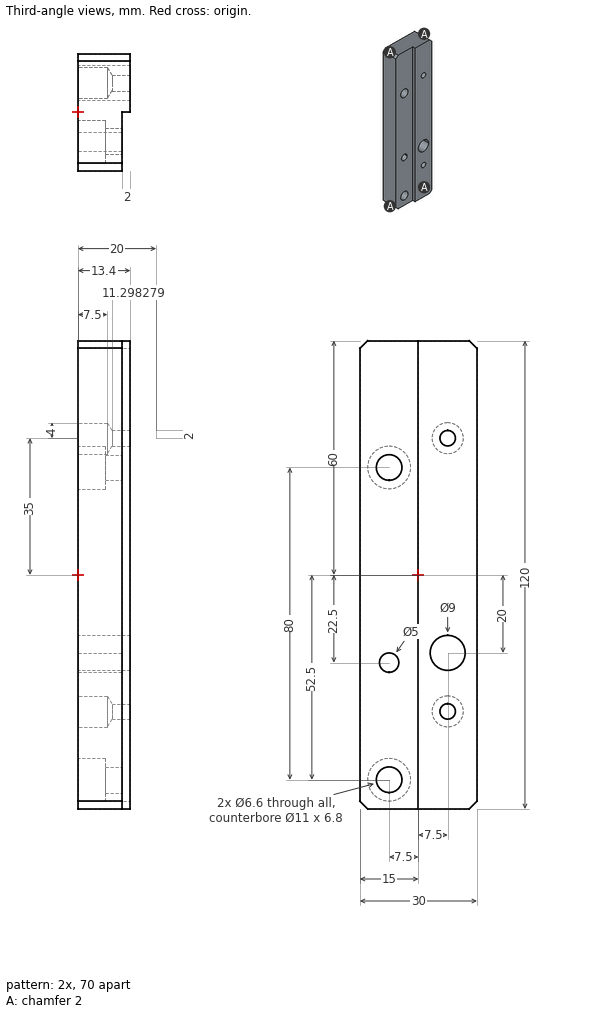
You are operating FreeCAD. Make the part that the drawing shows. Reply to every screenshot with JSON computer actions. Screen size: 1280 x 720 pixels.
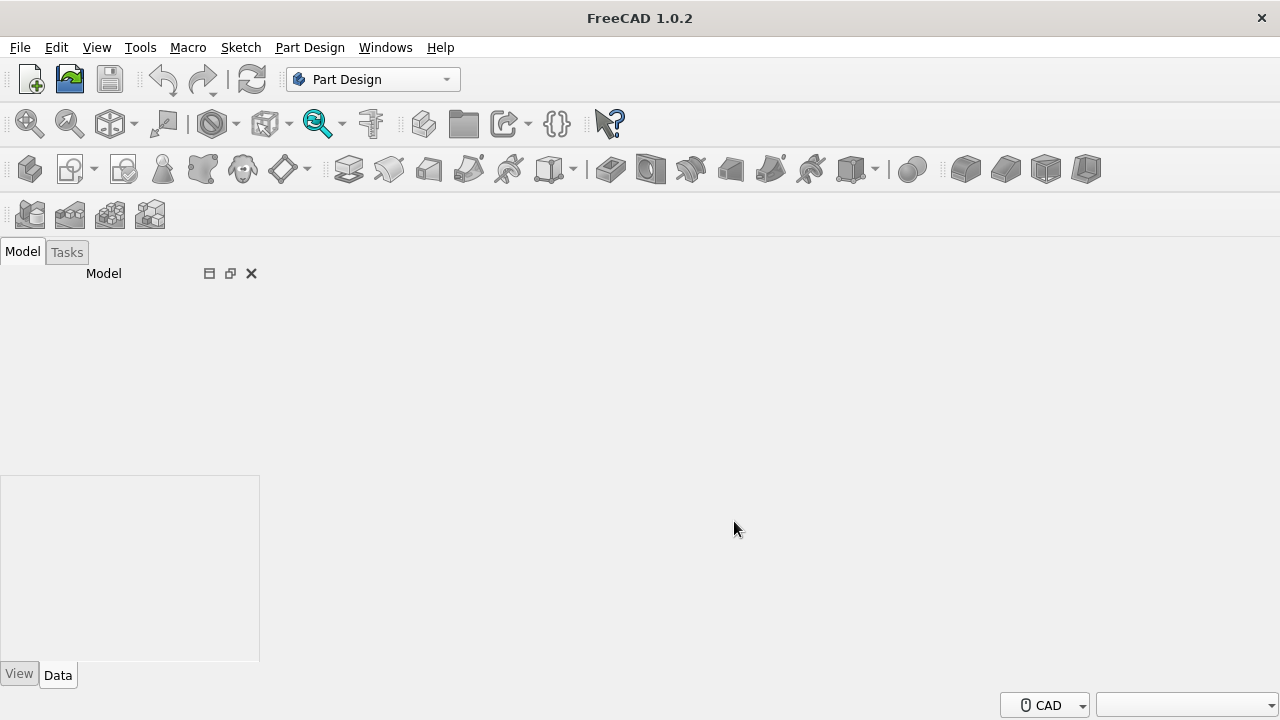
{"action": "left_click", "coordinate": [30, 80]}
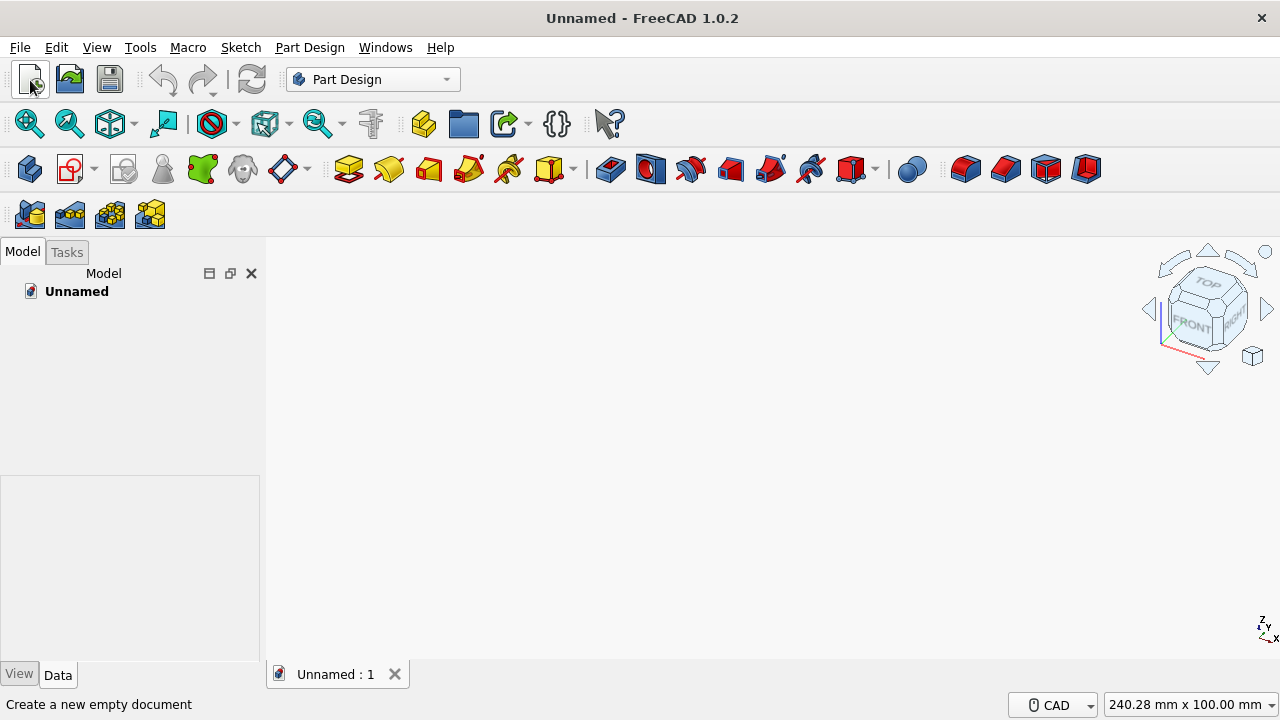
{"action": "left_click", "coordinate": [70, 170]}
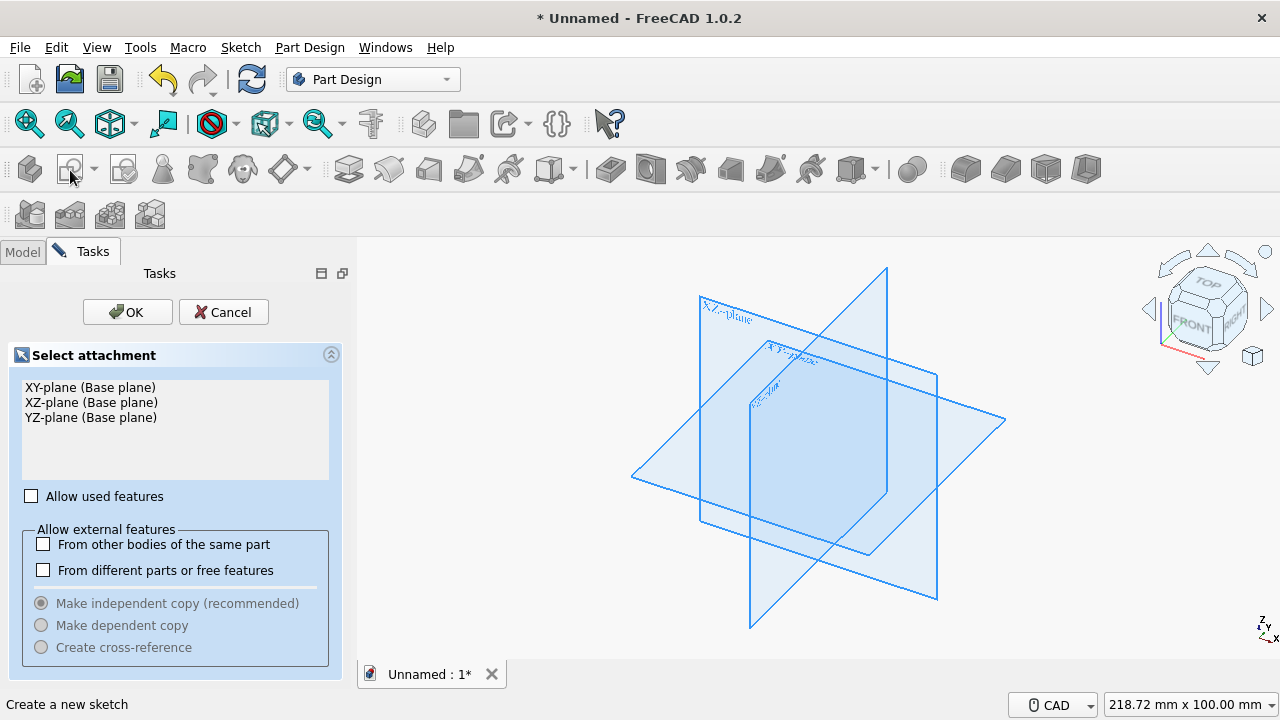
{"action": "left_click", "coordinate": [82, 418]}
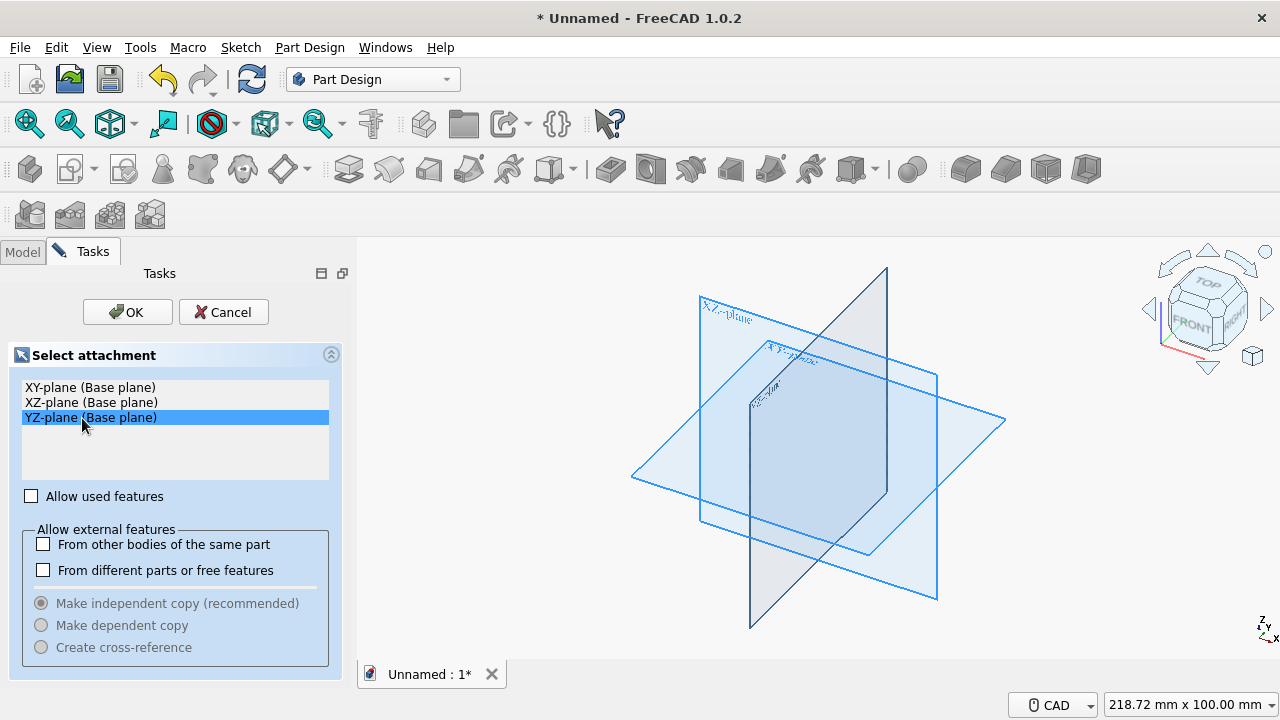
{"action": "left_click", "coordinate": [128, 312]}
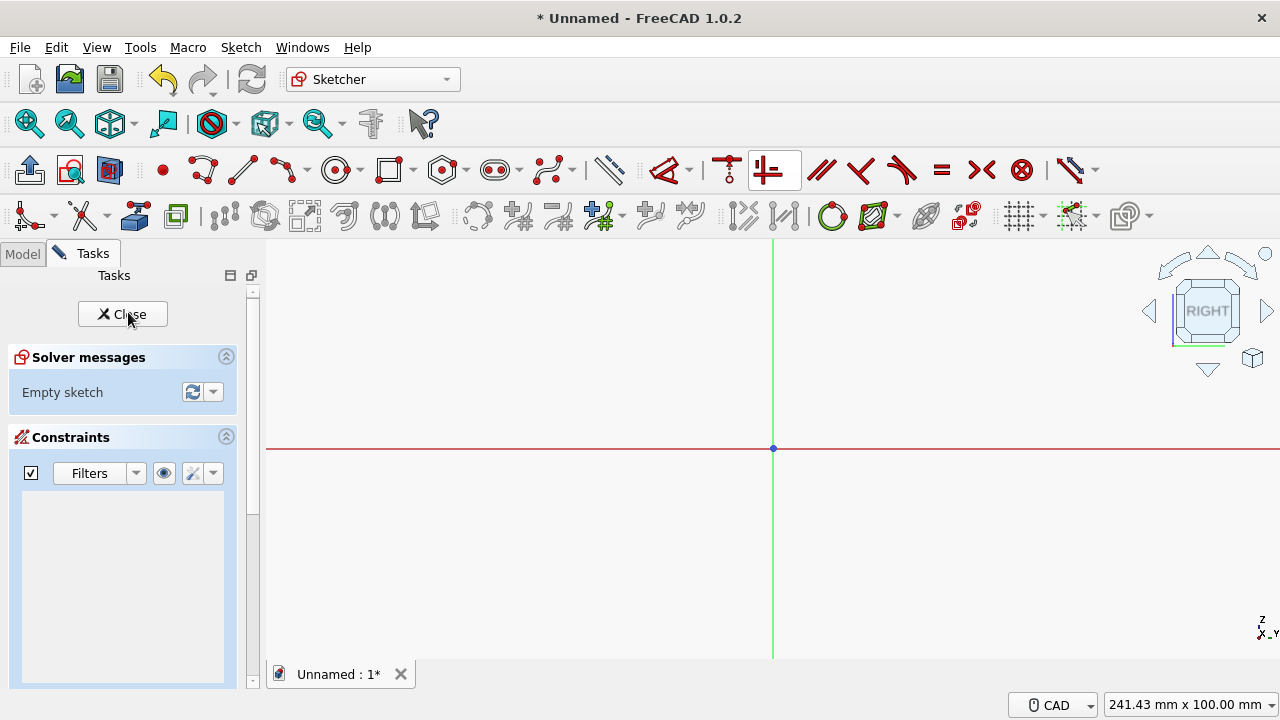
{"action": "scroll", "coordinate": [621, 449], "scroll_direction": "down", "scroll_amount": 3}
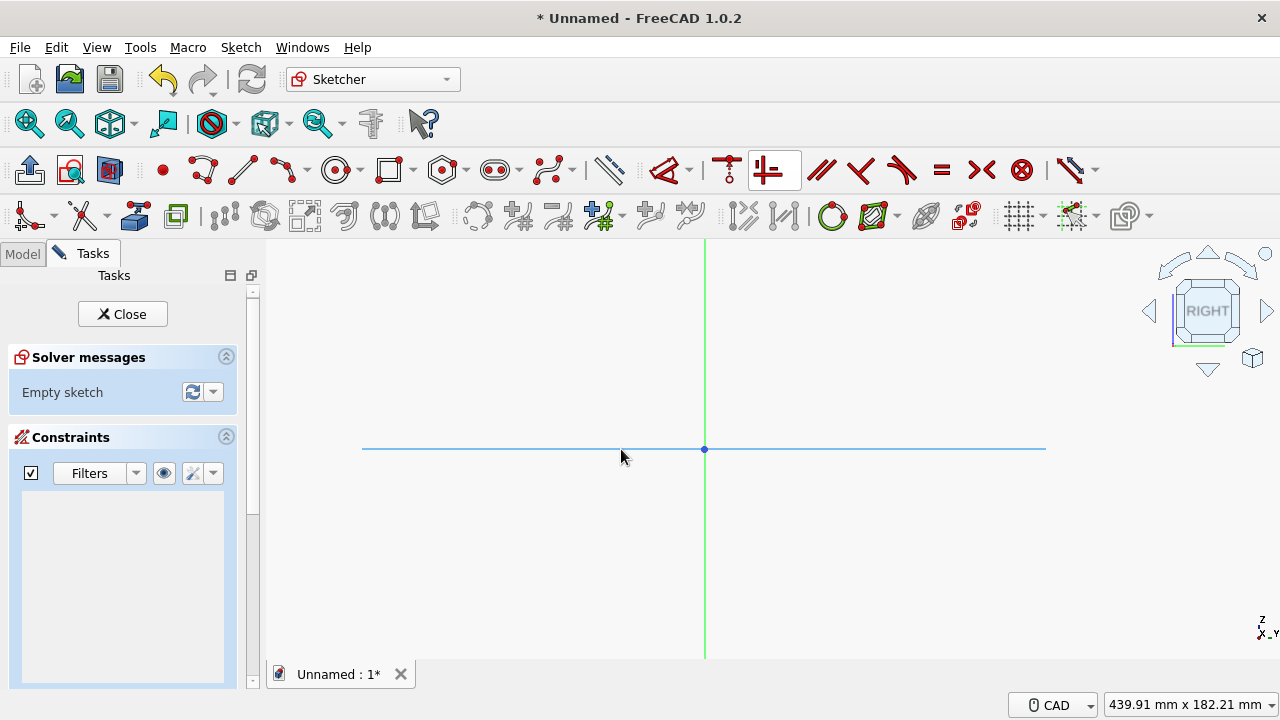
{"action": "left_click", "coordinate": [416, 170]}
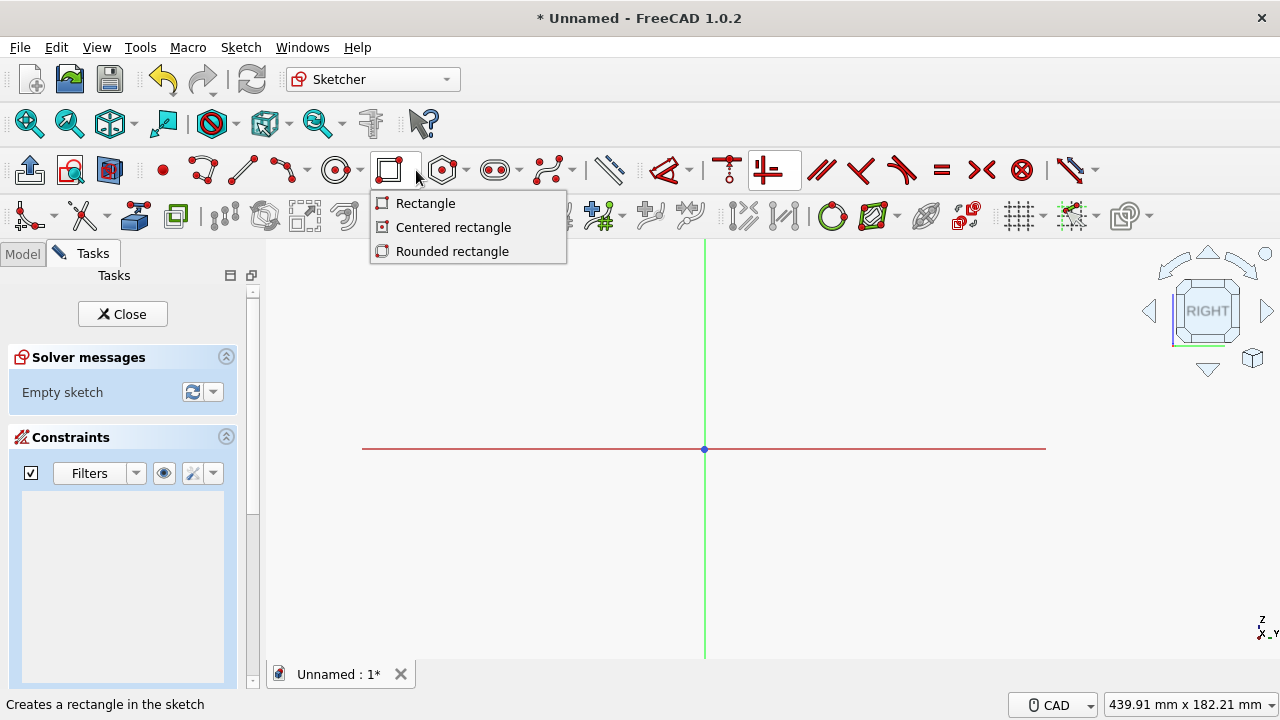
{"action": "left_click", "coordinate": [468, 227]}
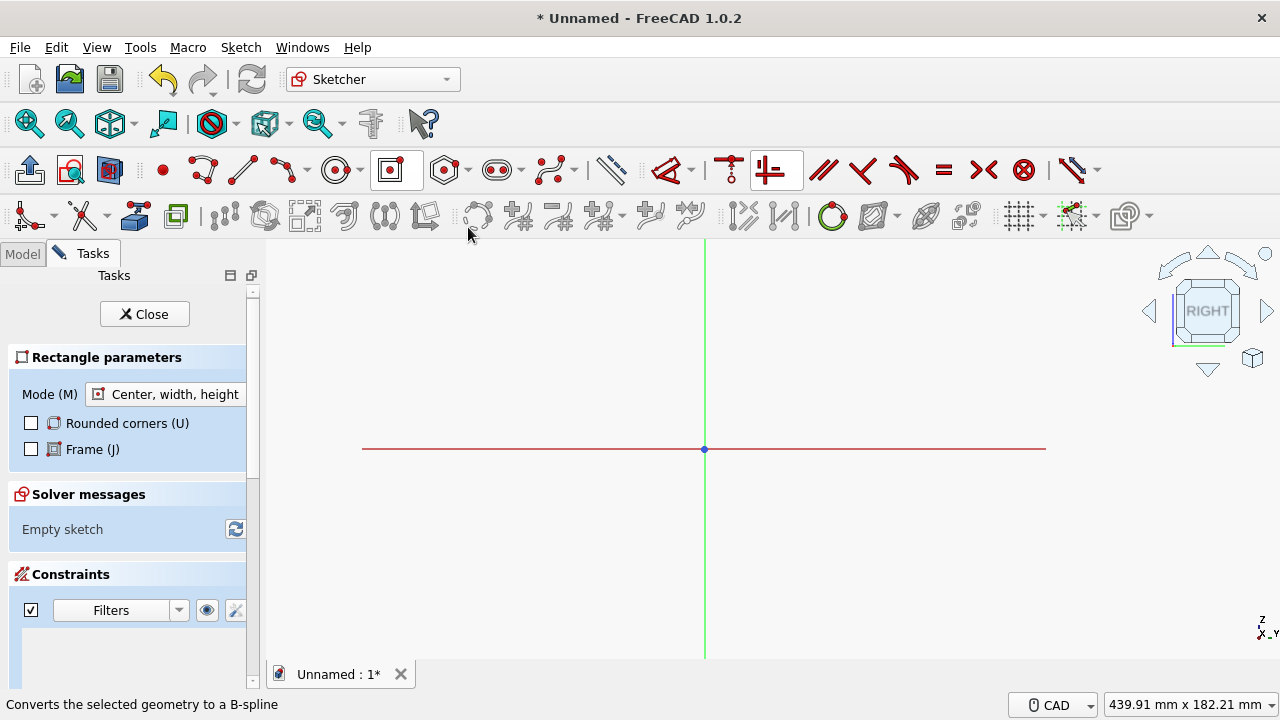
{"action": "left_click", "coordinate": [705, 449]}
{"action": "left_click", "coordinate": [739, 311]}
{"action": "key", "text": "Escape"}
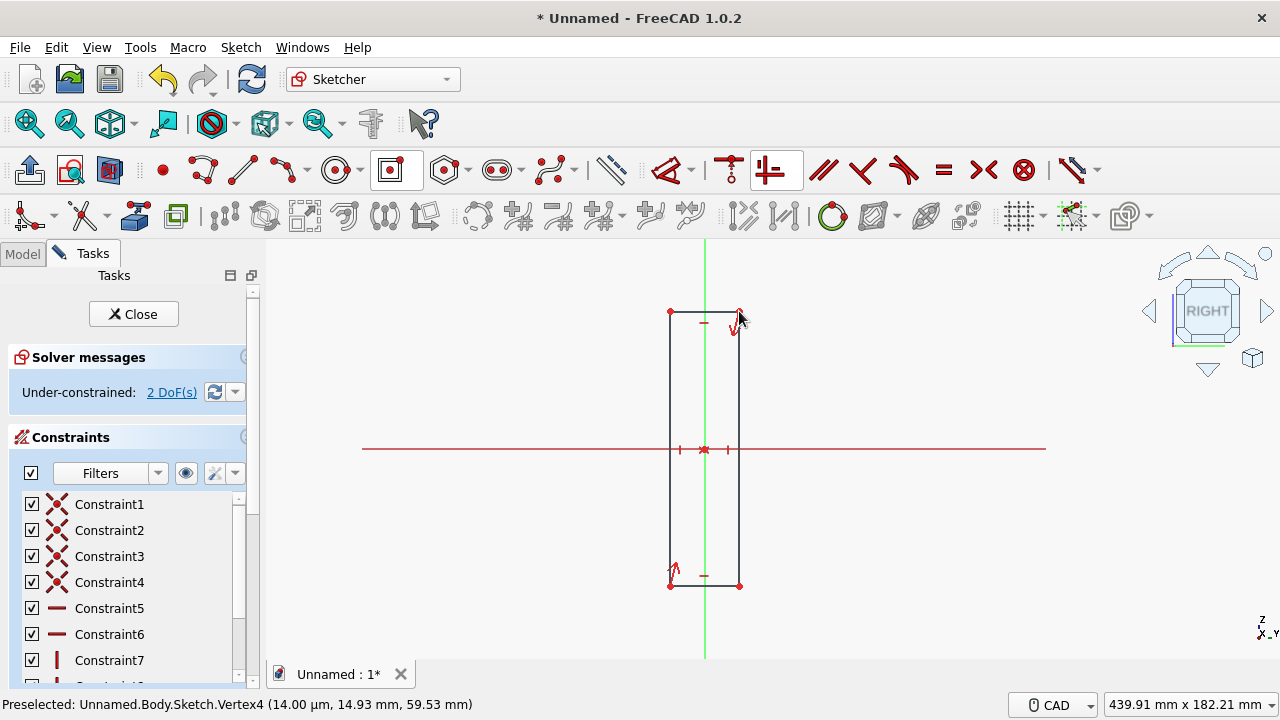
{"action": "left_click", "coordinate": [691, 586]}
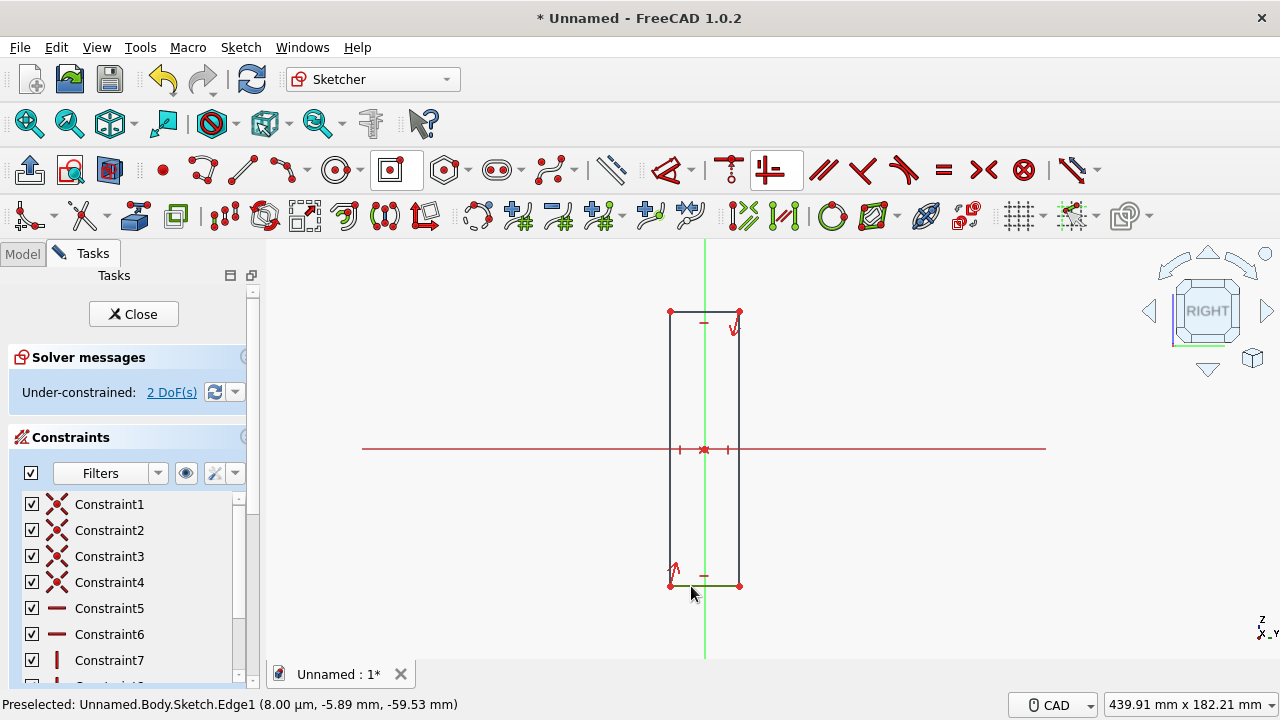
{"action": "left_click", "coordinate": [694, 170]}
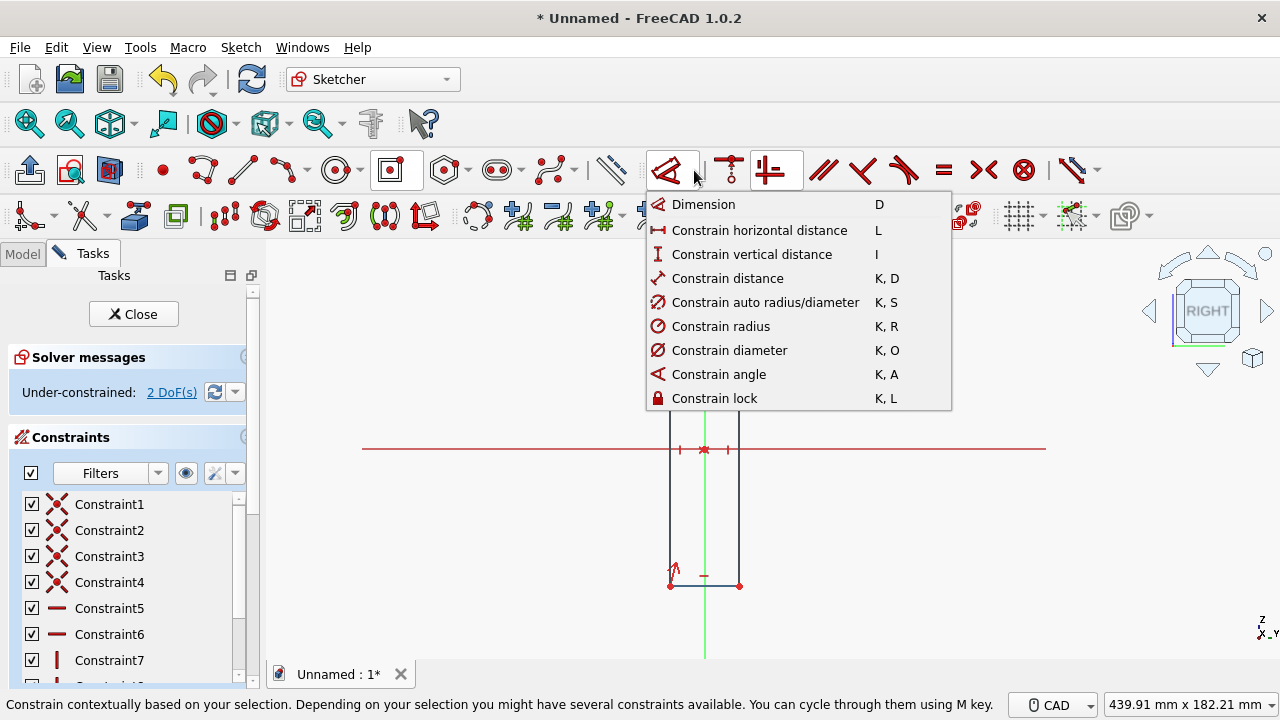
{"action": "left_click", "coordinate": [799, 230]}